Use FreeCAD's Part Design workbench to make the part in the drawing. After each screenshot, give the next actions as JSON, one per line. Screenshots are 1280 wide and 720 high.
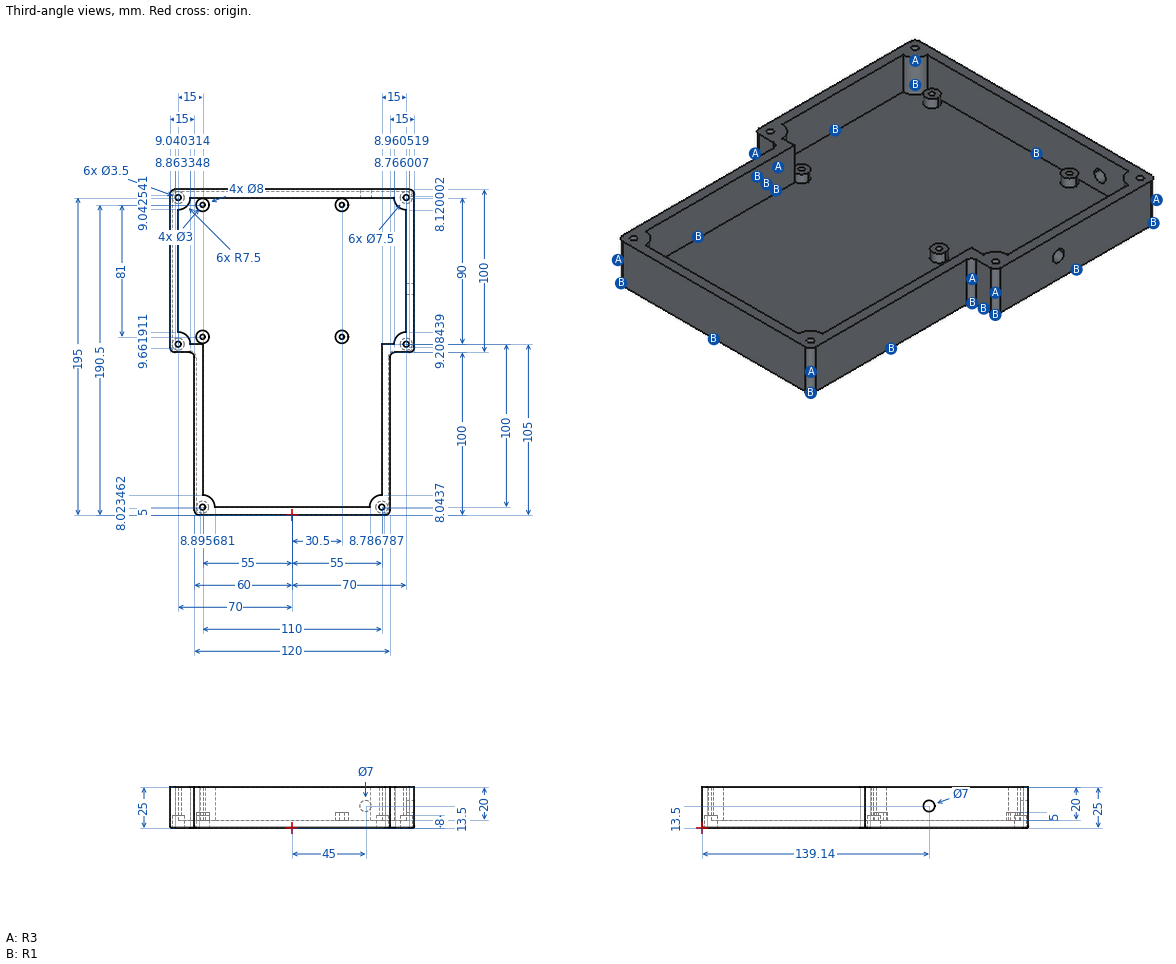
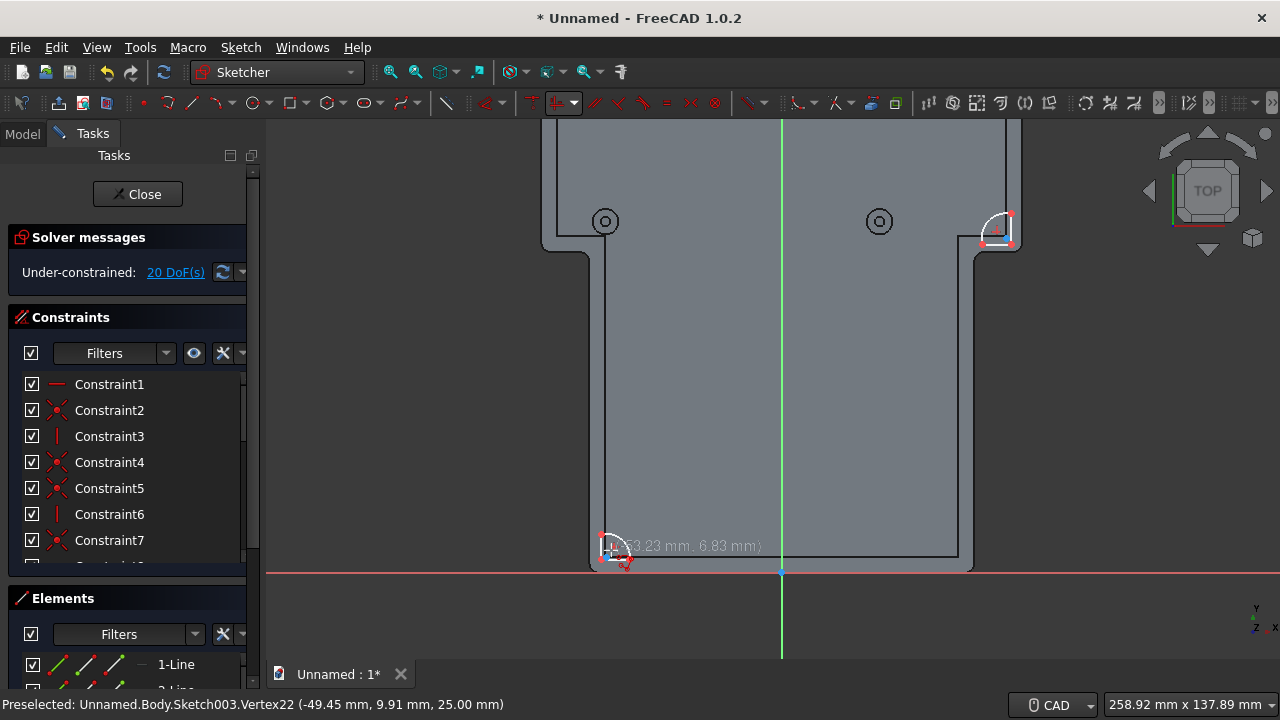
{"action": "scroll", "coordinate": [789, 555], "scroll_direction": "up", "scroll_amount": 4}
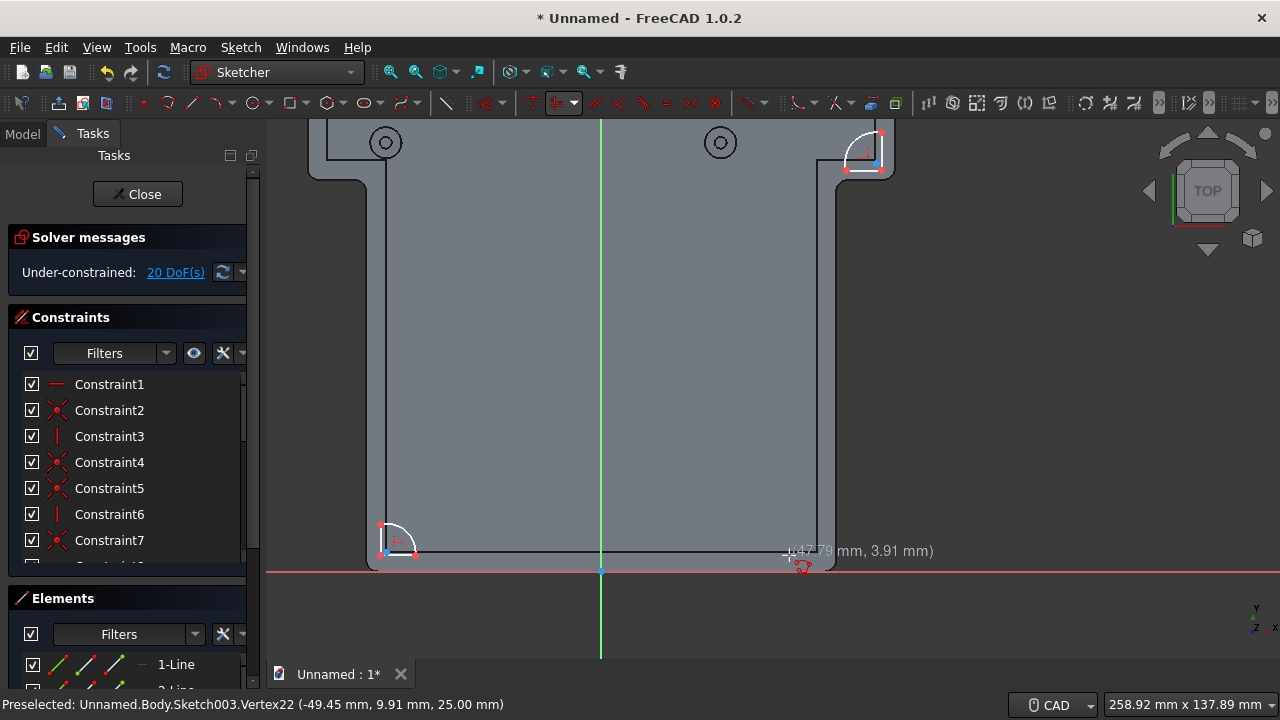
{"action": "left_click", "coordinate": [787, 555]}
{"action": "left_click", "coordinate": [822, 555]}
{"action": "left_click", "coordinate": [822, 523]}
{"action": "right_click", "coordinate": [822, 523]}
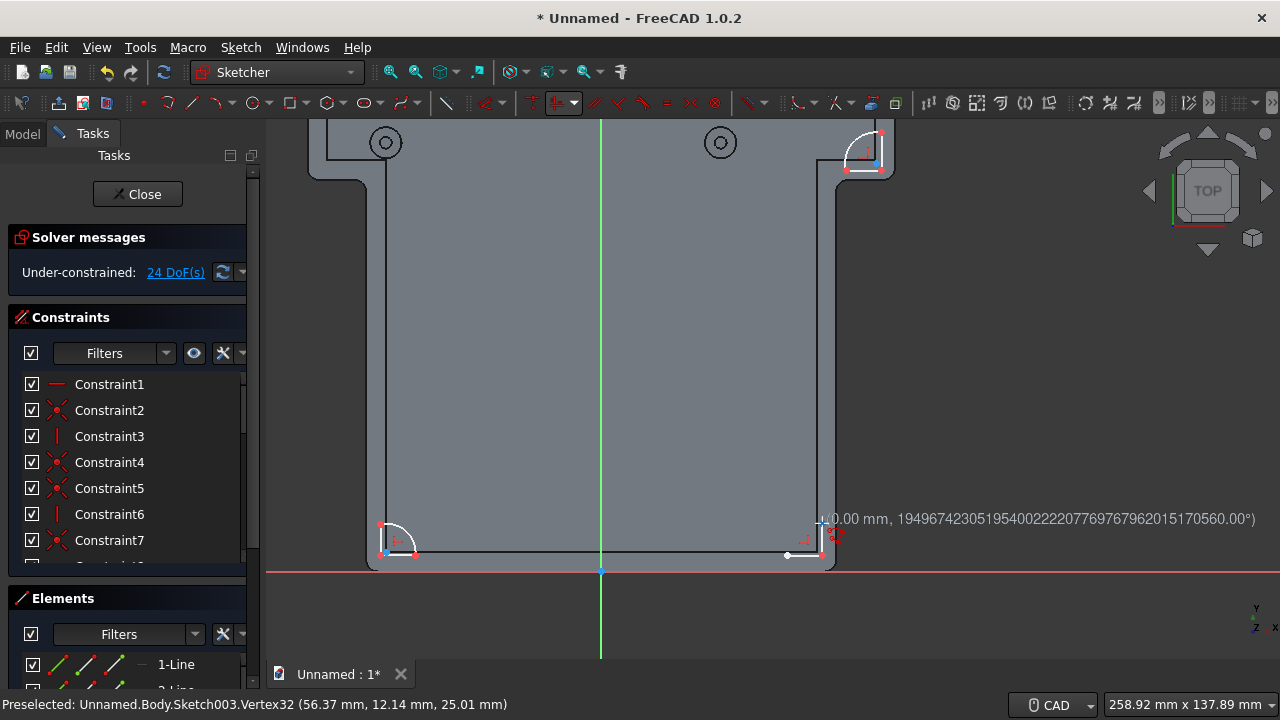
{"action": "key", "text": "g 3 a"}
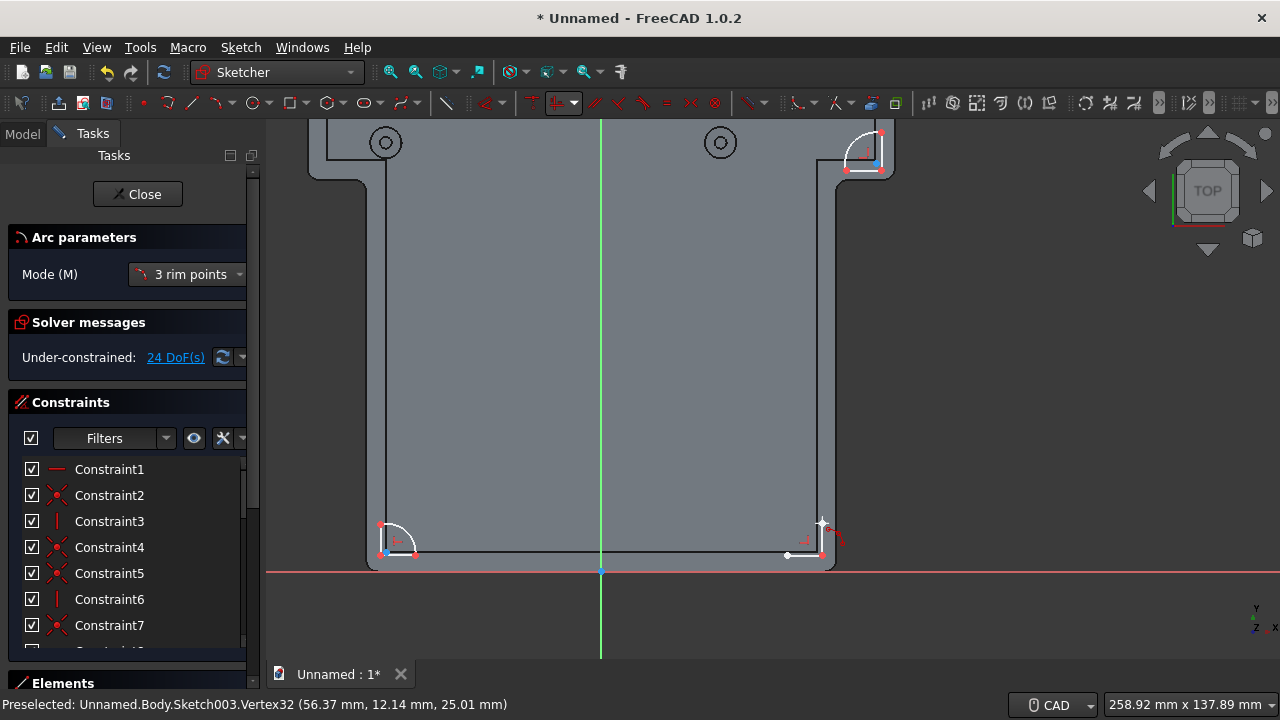
{"action": "left_click", "coordinate": [822, 524]}
{"action": "left_click", "coordinate": [787, 556]}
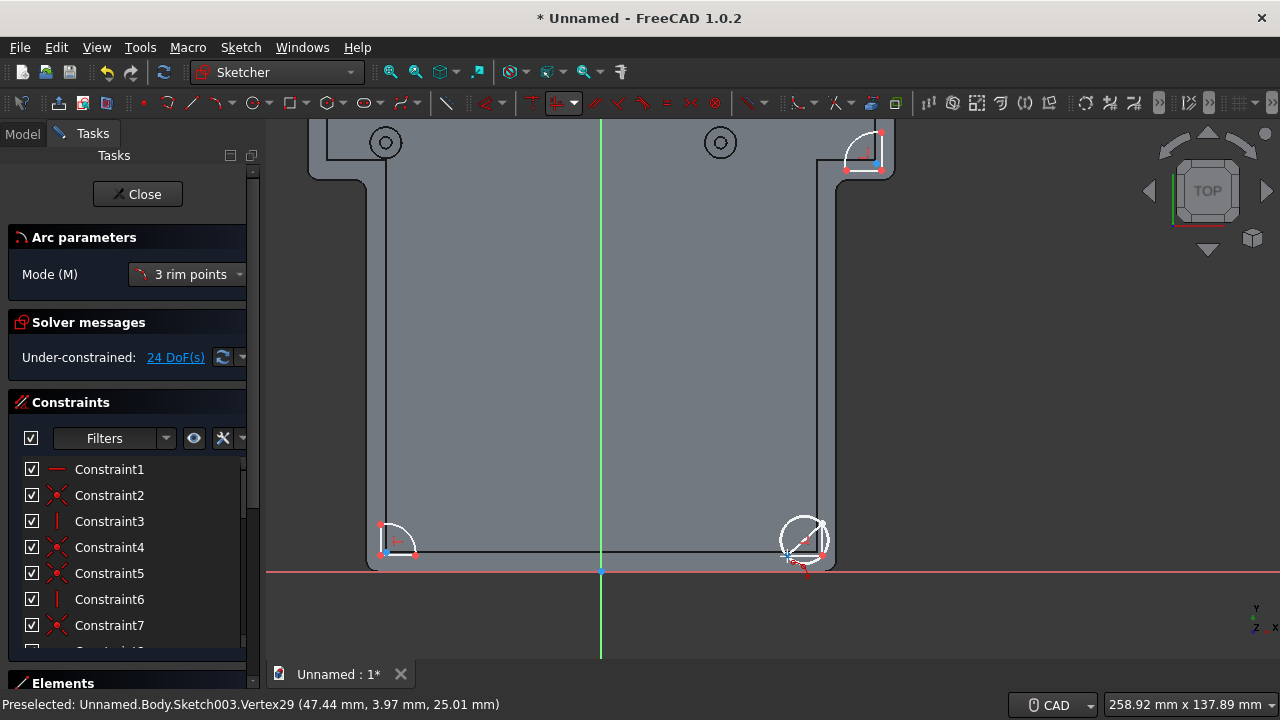
{"action": "scroll", "coordinate": [797, 530], "scroll_direction": "up", "scroll_amount": 2}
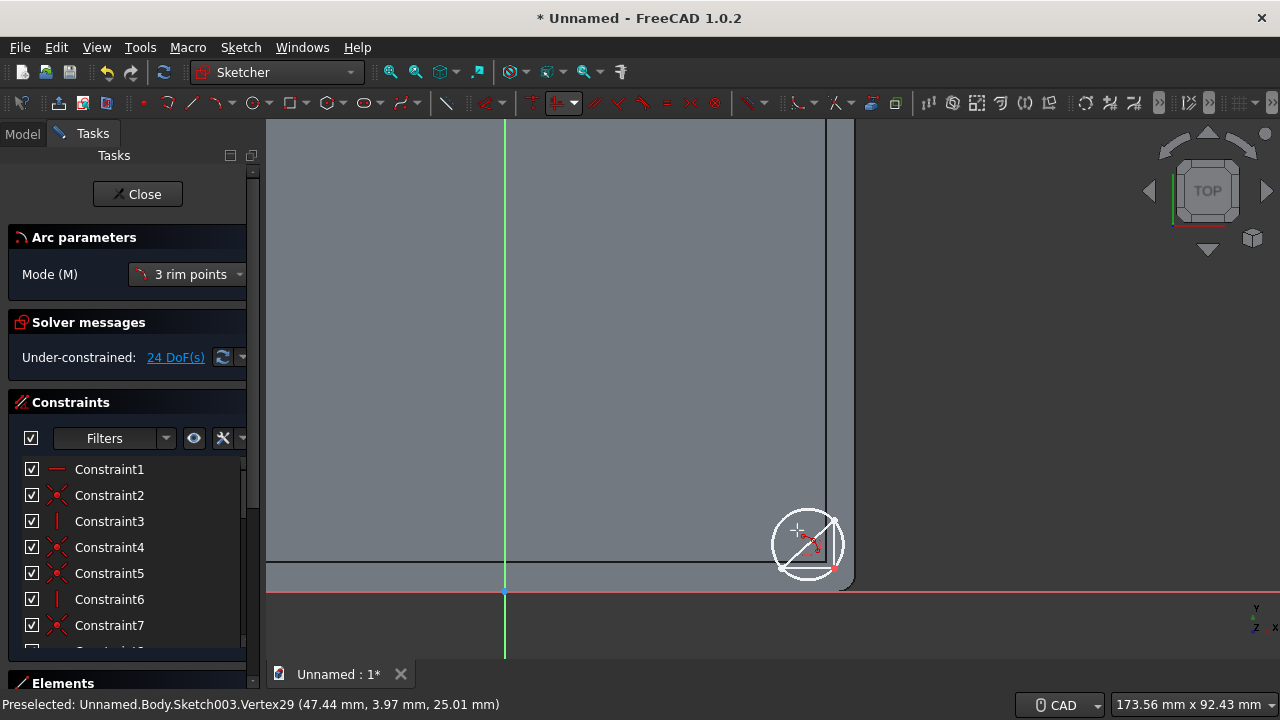
{"action": "left_click", "coordinate": [796, 530]}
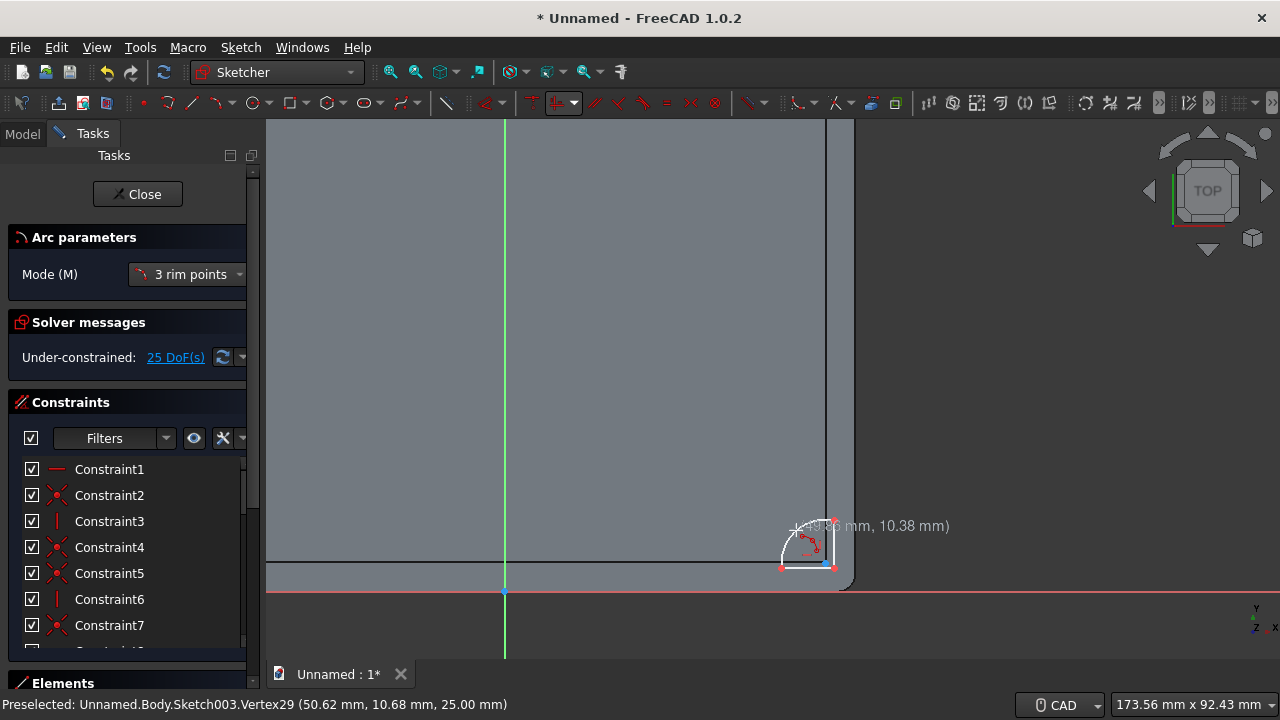
{"action": "key", "text": "g m"}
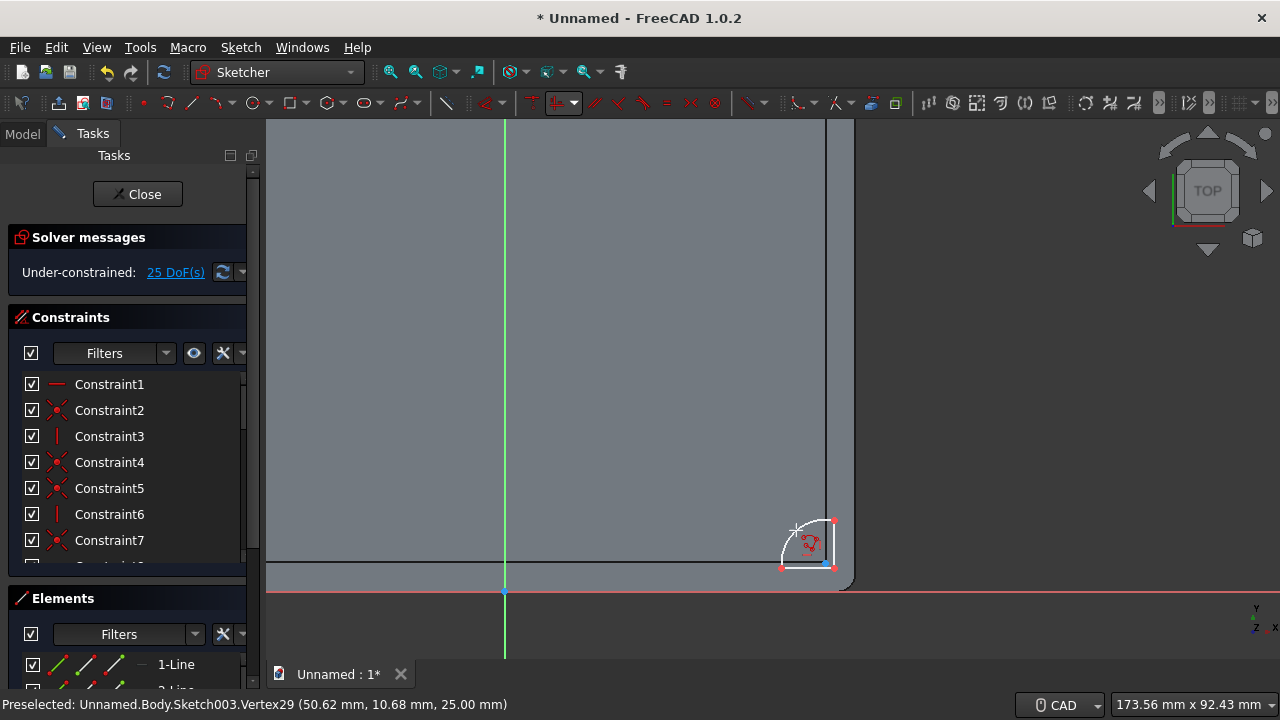
{"action": "scroll", "coordinate": [791, 549], "scroll_direction": "down", "scroll_amount": 6}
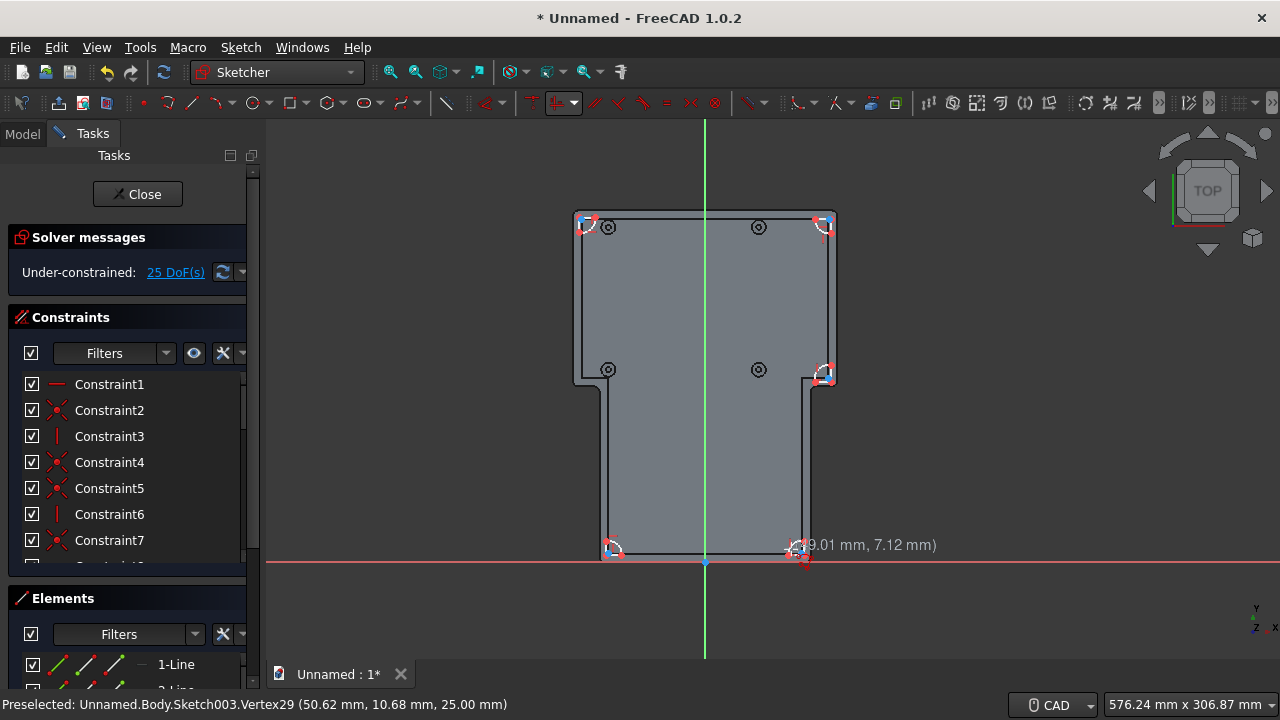
{"action": "left_click", "coordinate": [579, 365]}
{"action": "left_click", "coordinate": [579, 382]}
{"action": "left_click", "coordinate": [594, 382]}
{"action": "right_click", "coordinate": [594, 382]}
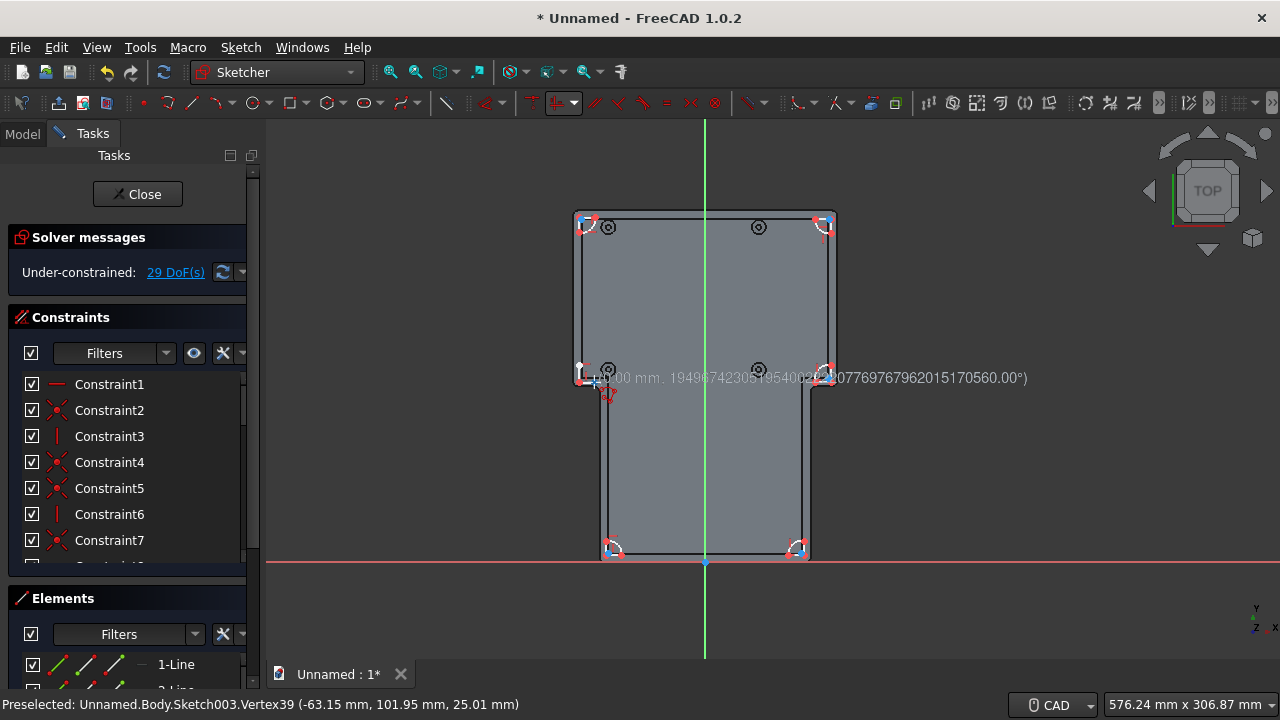
{"action": "left_click", "coordinate": [216, 104]}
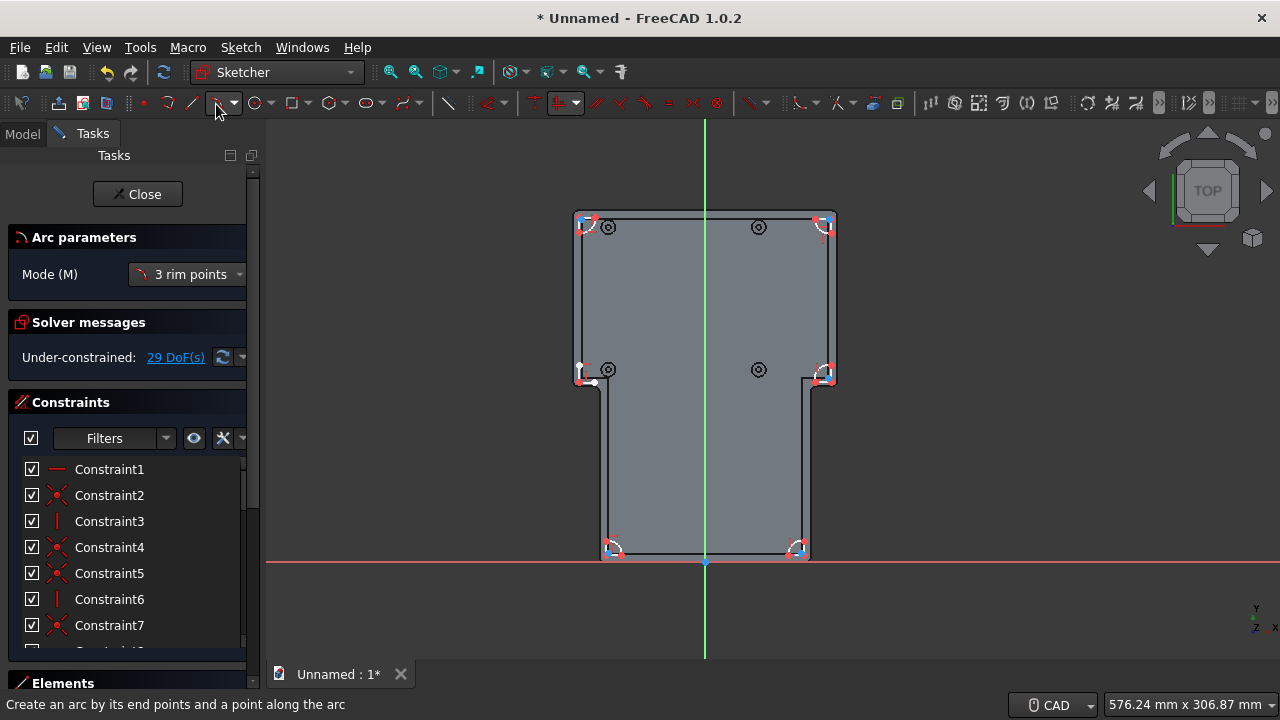
{"action": "scroll", "coordinate": [594, 382], "scroll_direction": "up", "scroll_amount": 4}